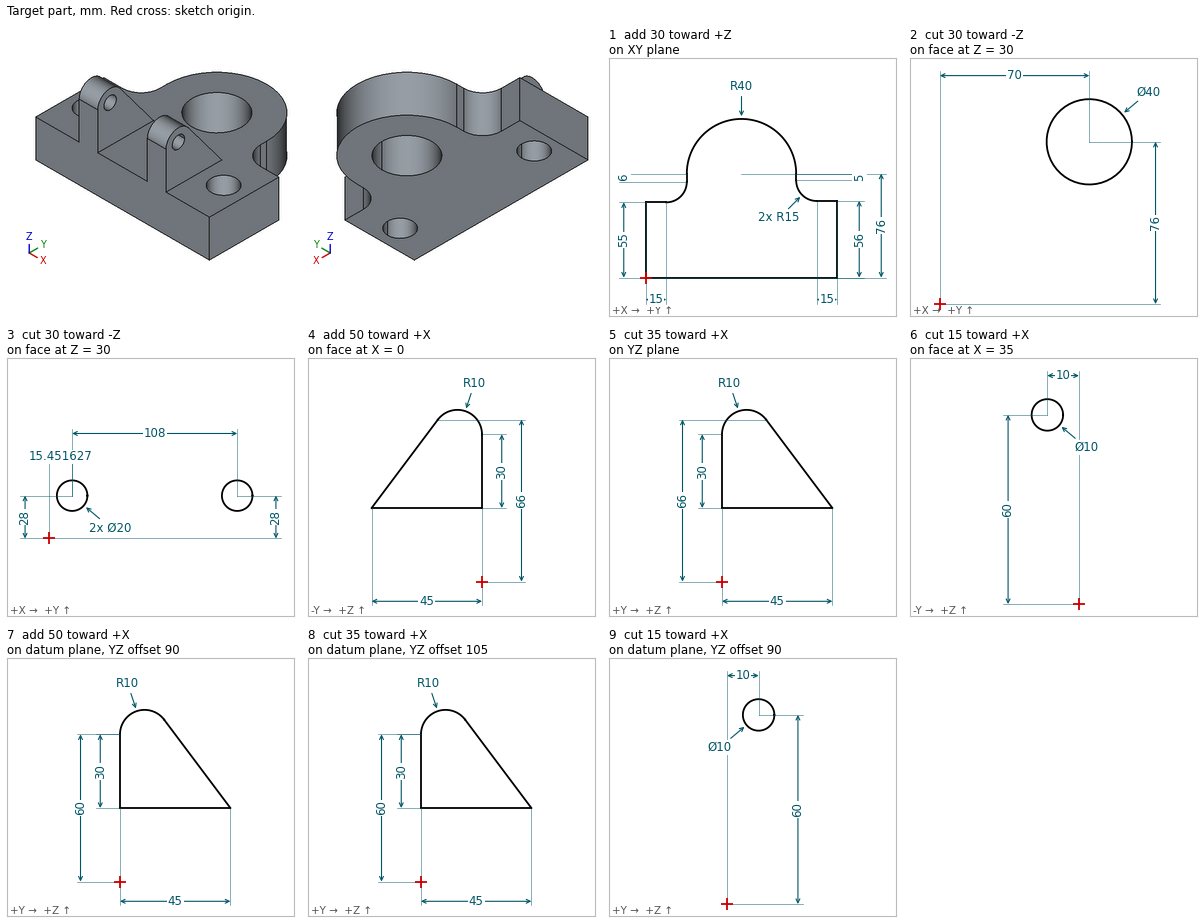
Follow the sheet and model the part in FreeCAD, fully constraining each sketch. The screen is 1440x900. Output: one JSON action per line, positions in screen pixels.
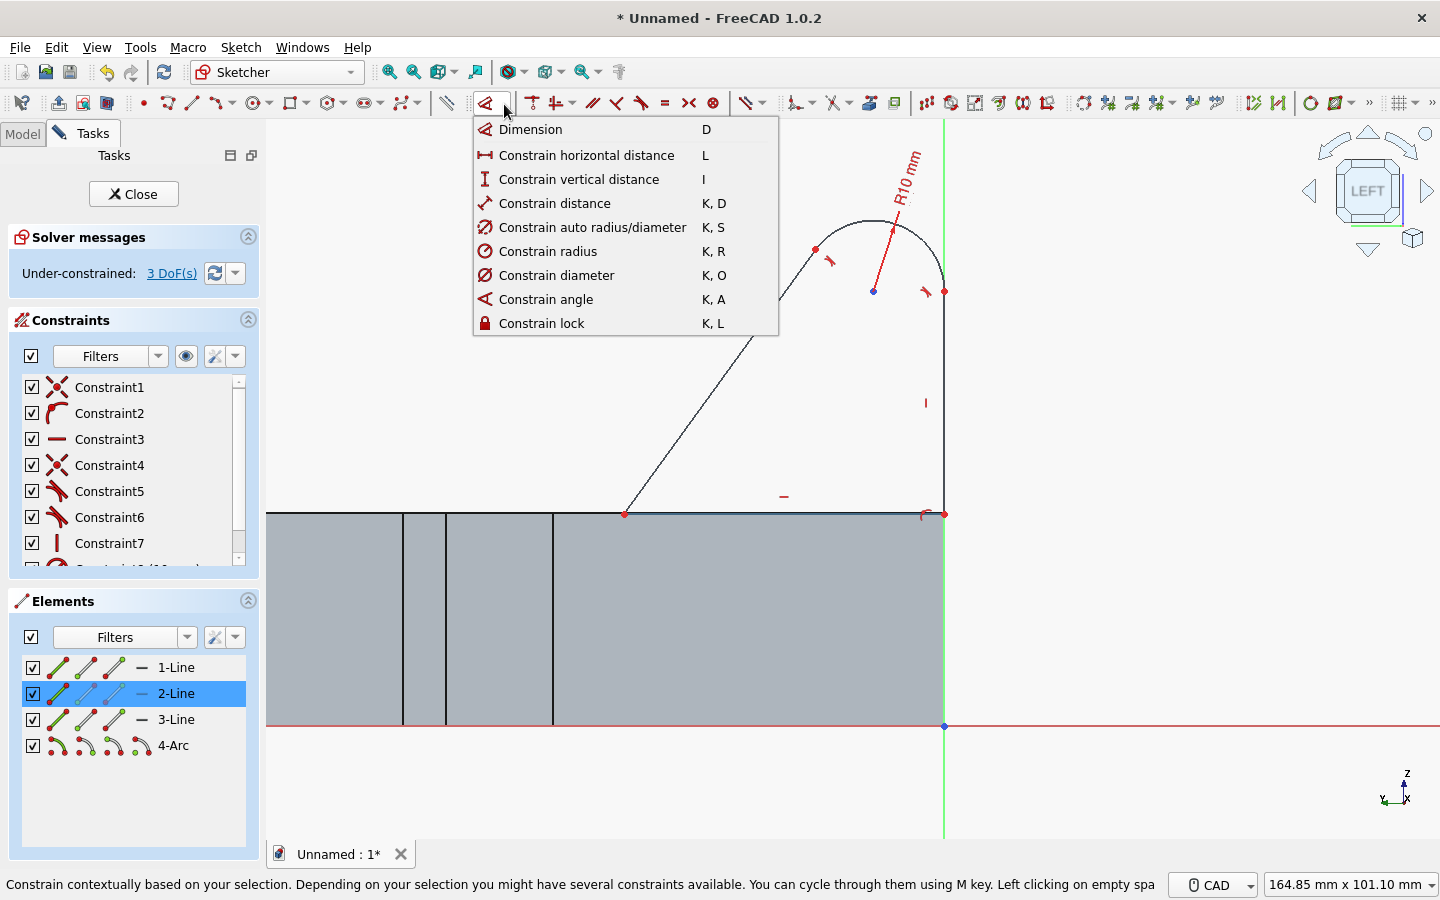
{"action": "left_click", "coordinate": [626, 155]}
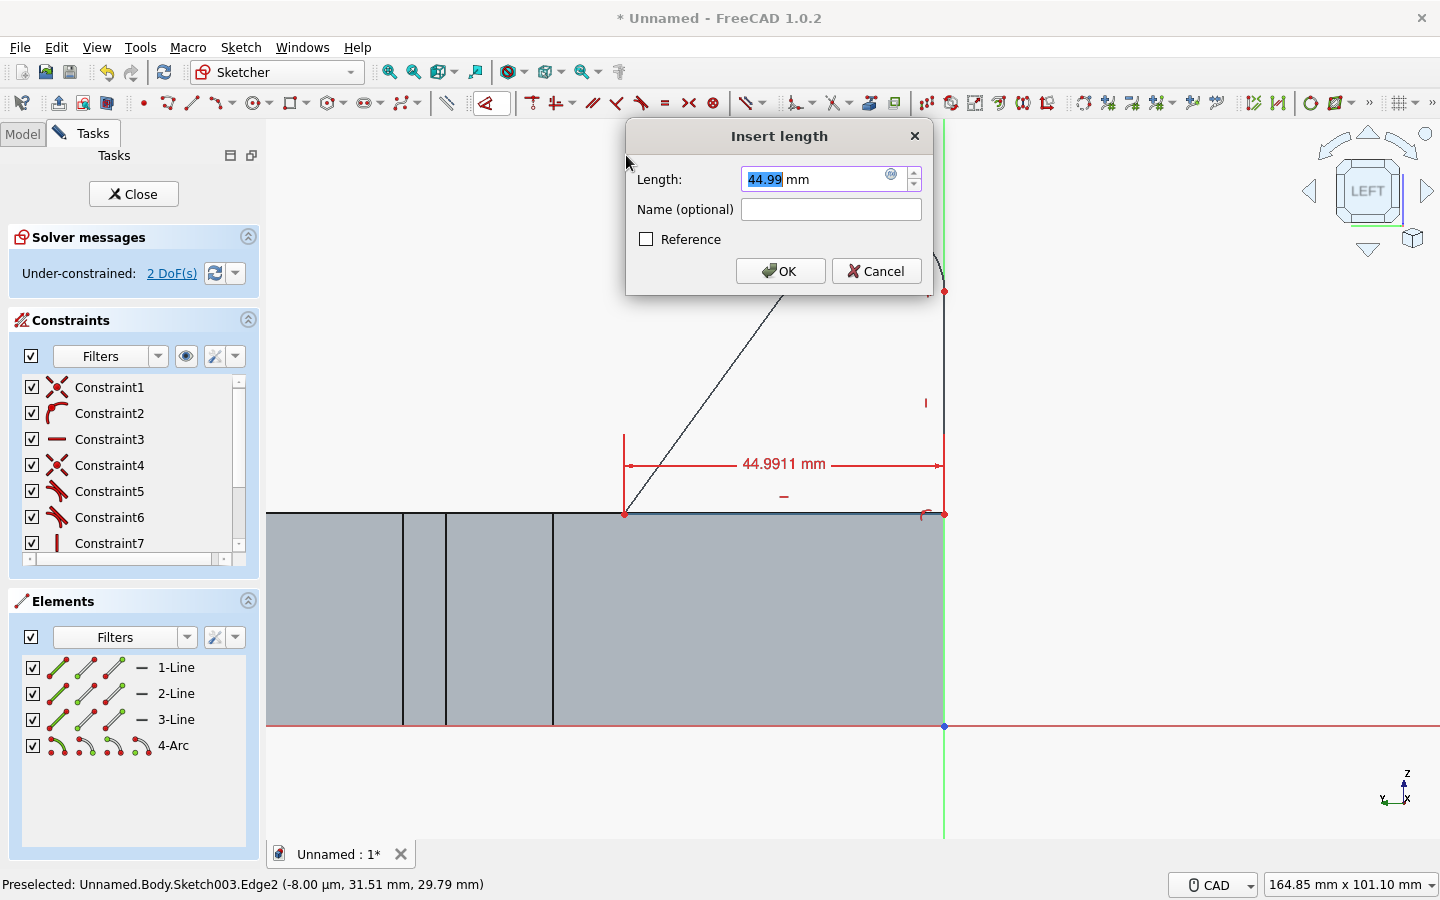
{"action": "type", "text": "45"}
{"action": "key", "text": "Return"}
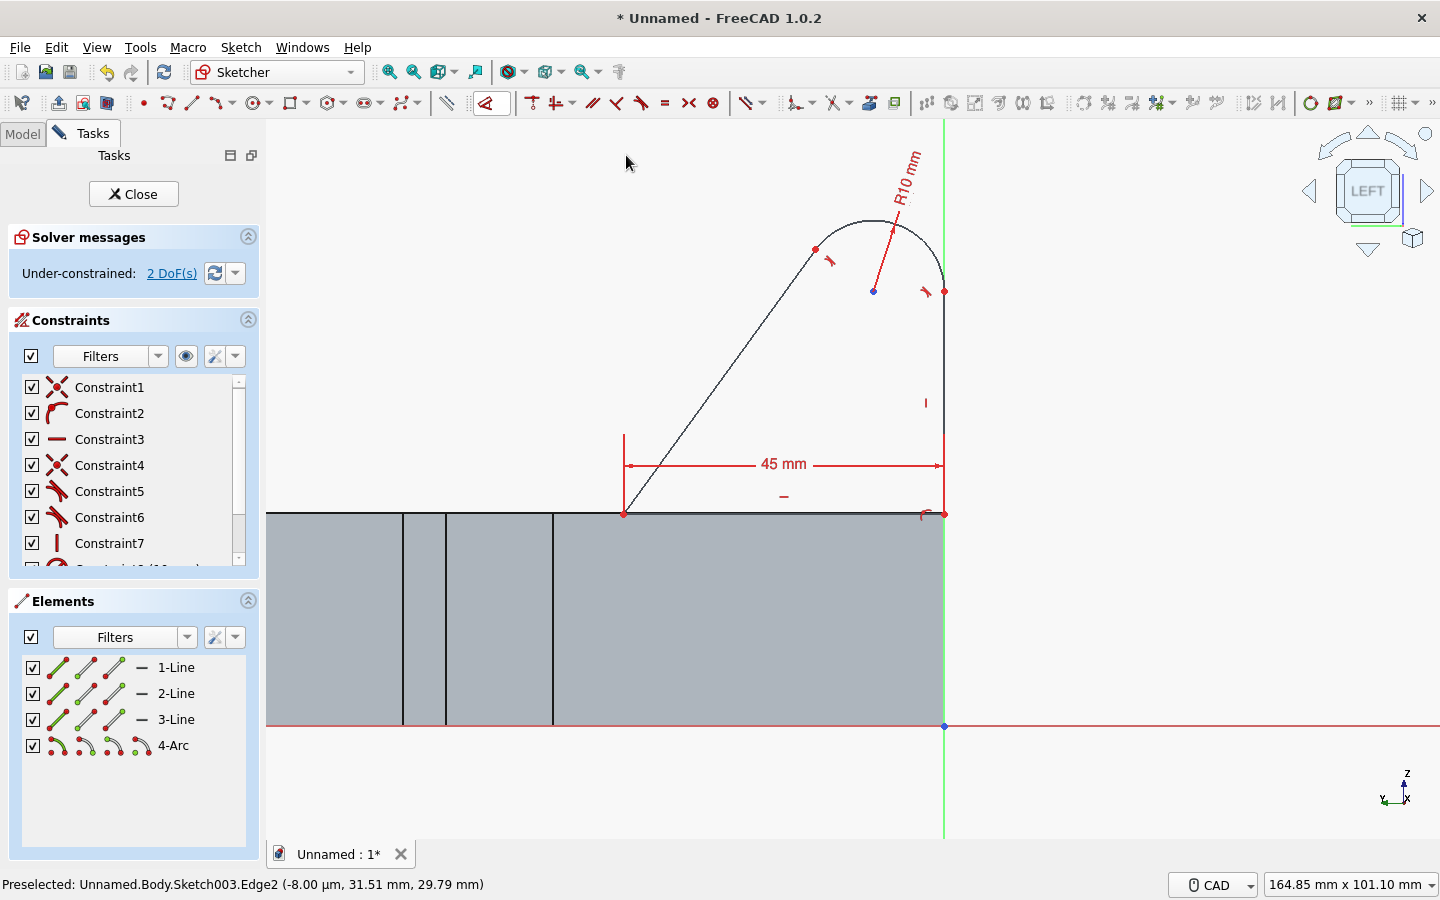
{"action": "left_click", "coordinate": [944, 447]}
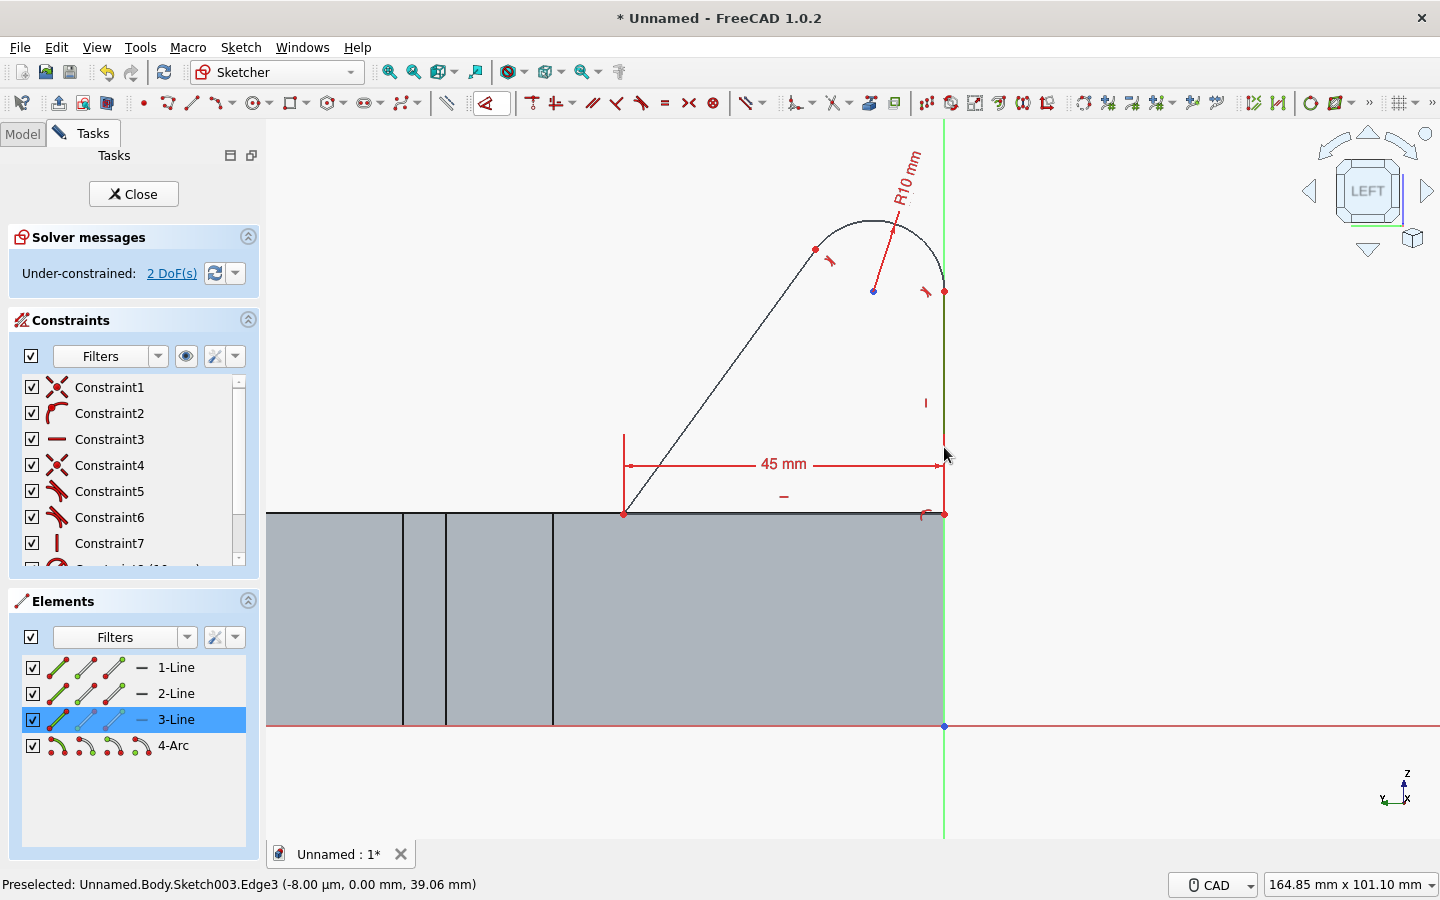
{"action": "key", "text": "i"}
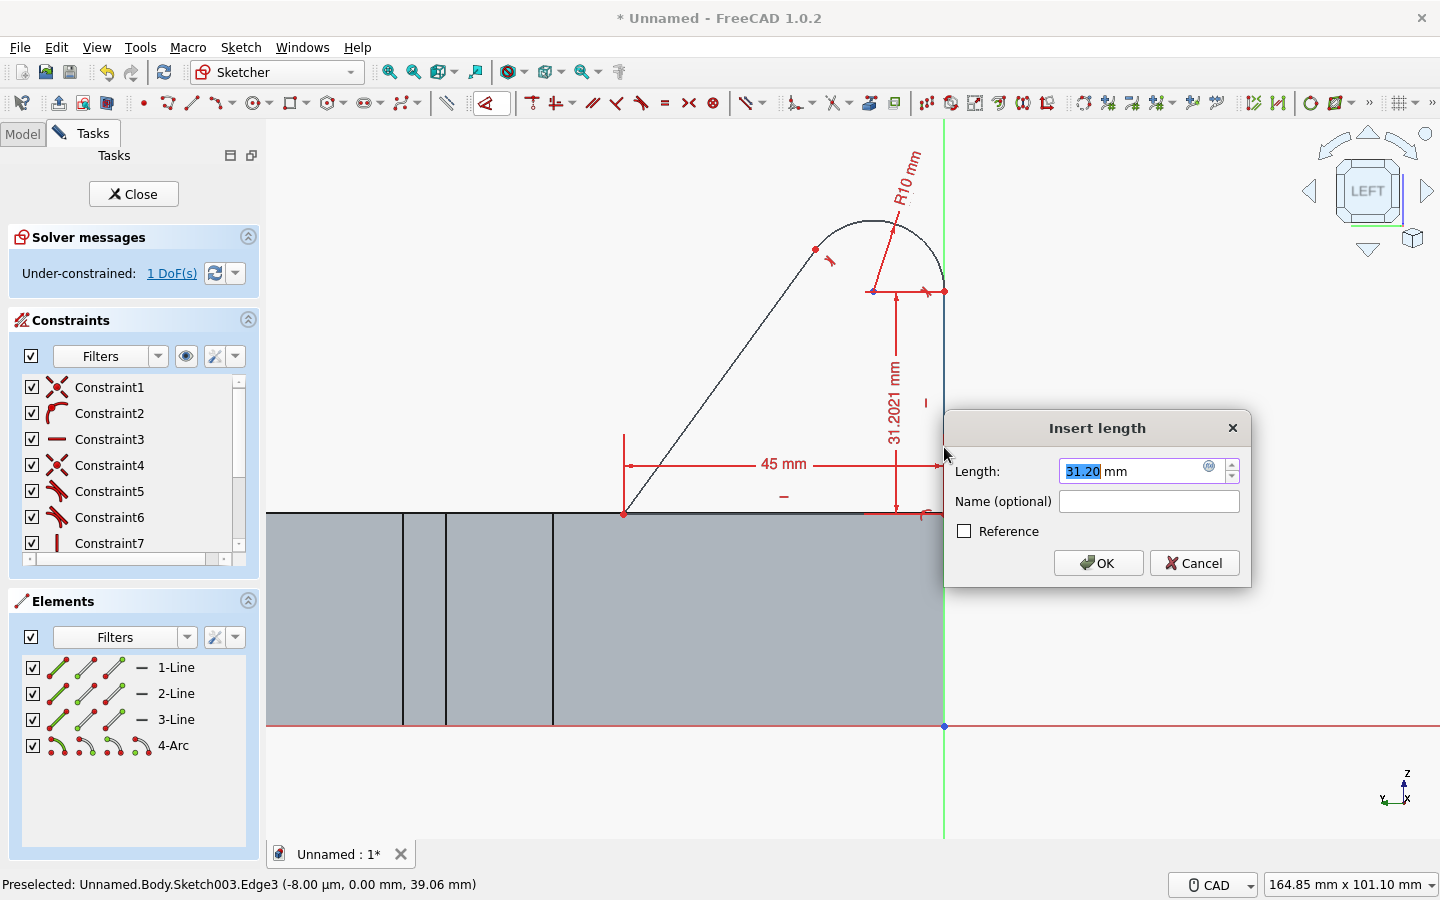
{"action": "type", "text": "30"}
{"action": "key", "text": "Return"}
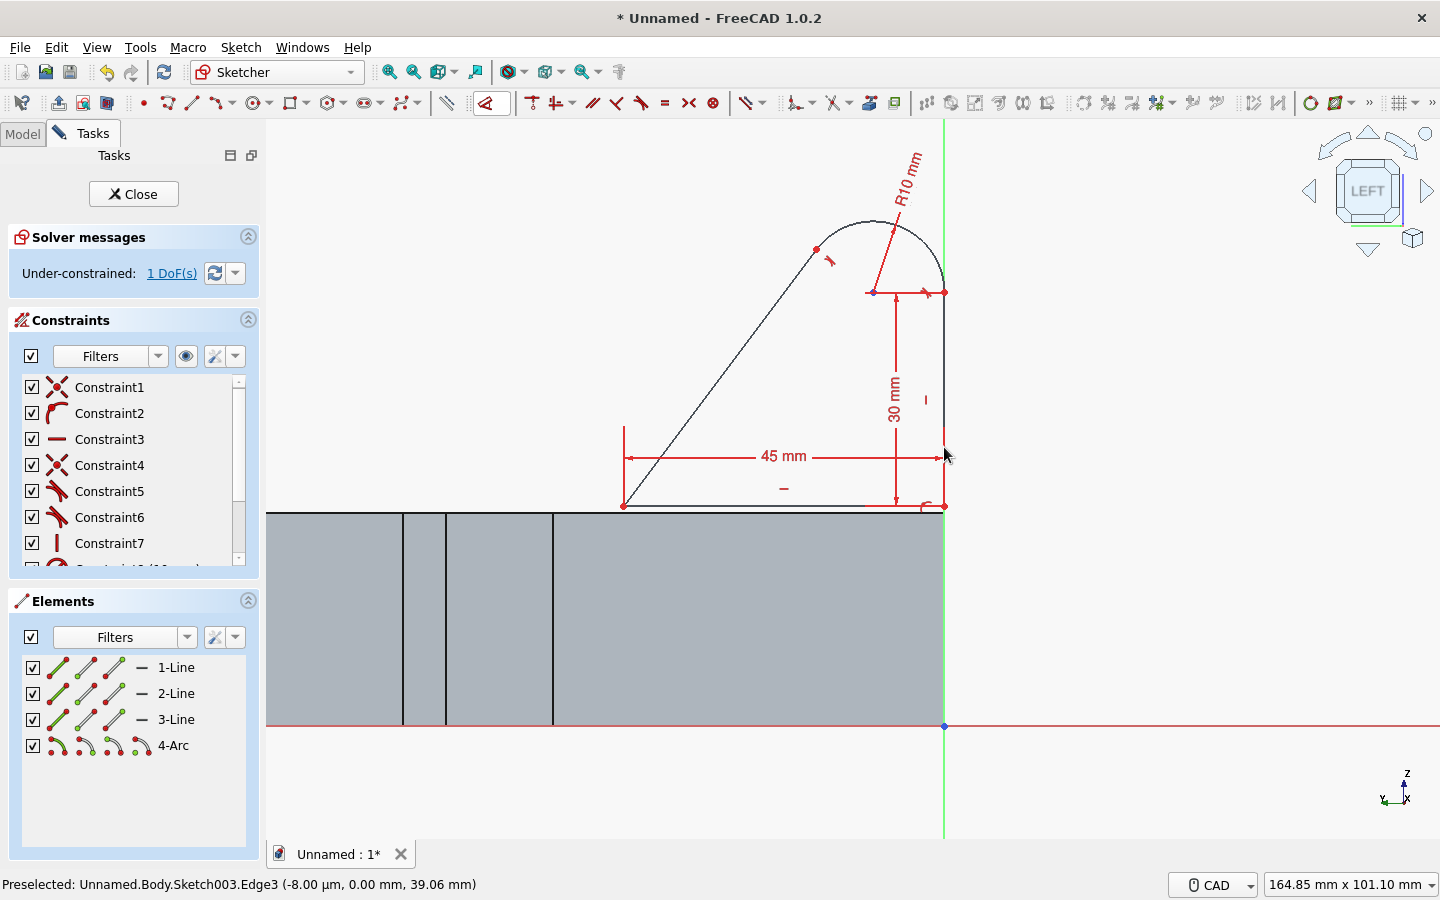
{"action": "left_click", "coordinate": [816, 250]}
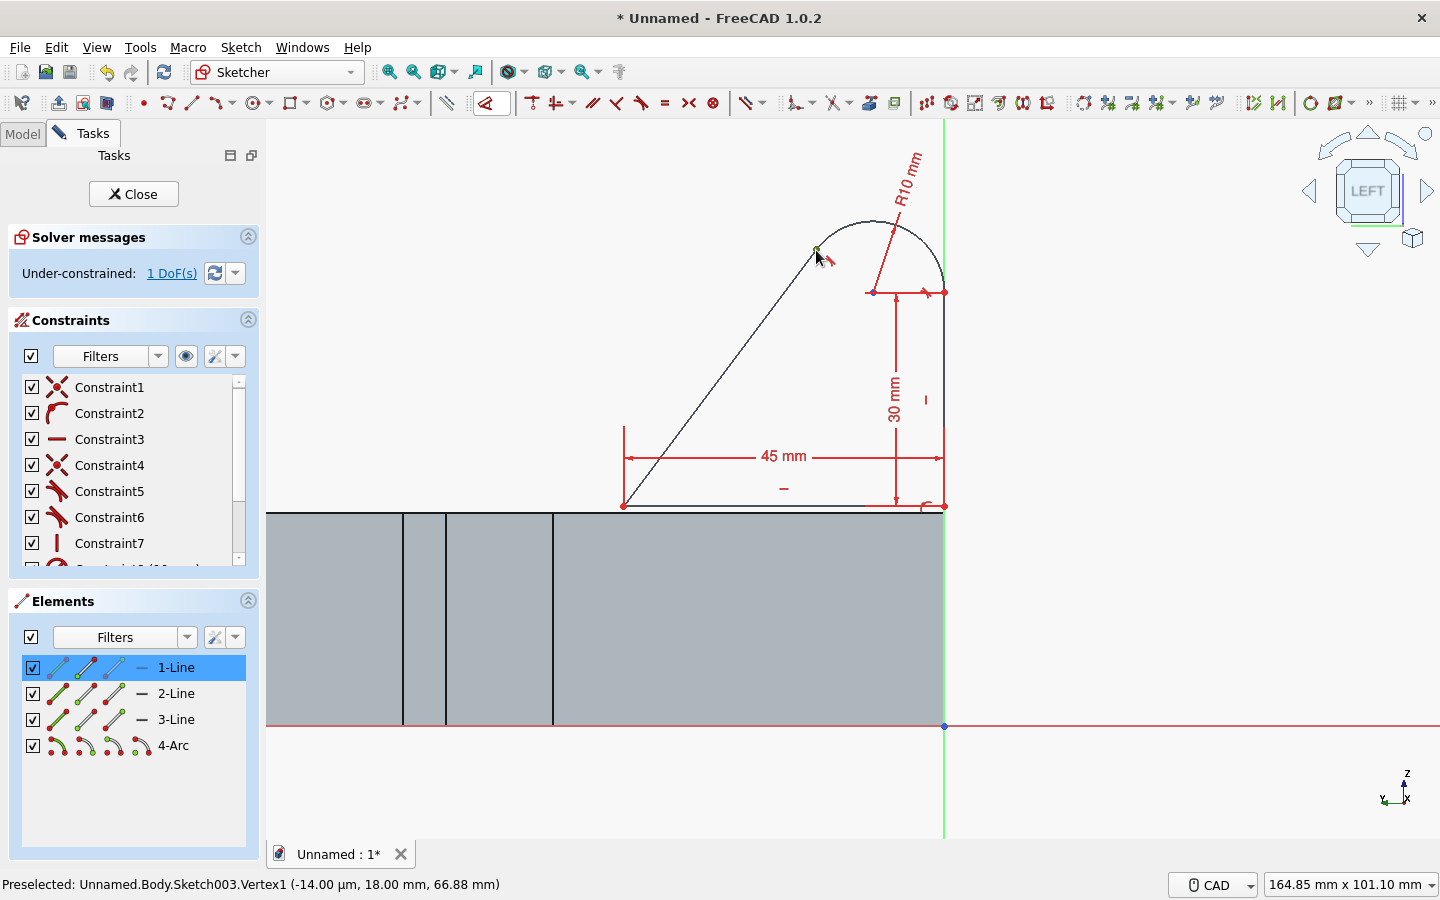
{"action": "key", "text": "i"}